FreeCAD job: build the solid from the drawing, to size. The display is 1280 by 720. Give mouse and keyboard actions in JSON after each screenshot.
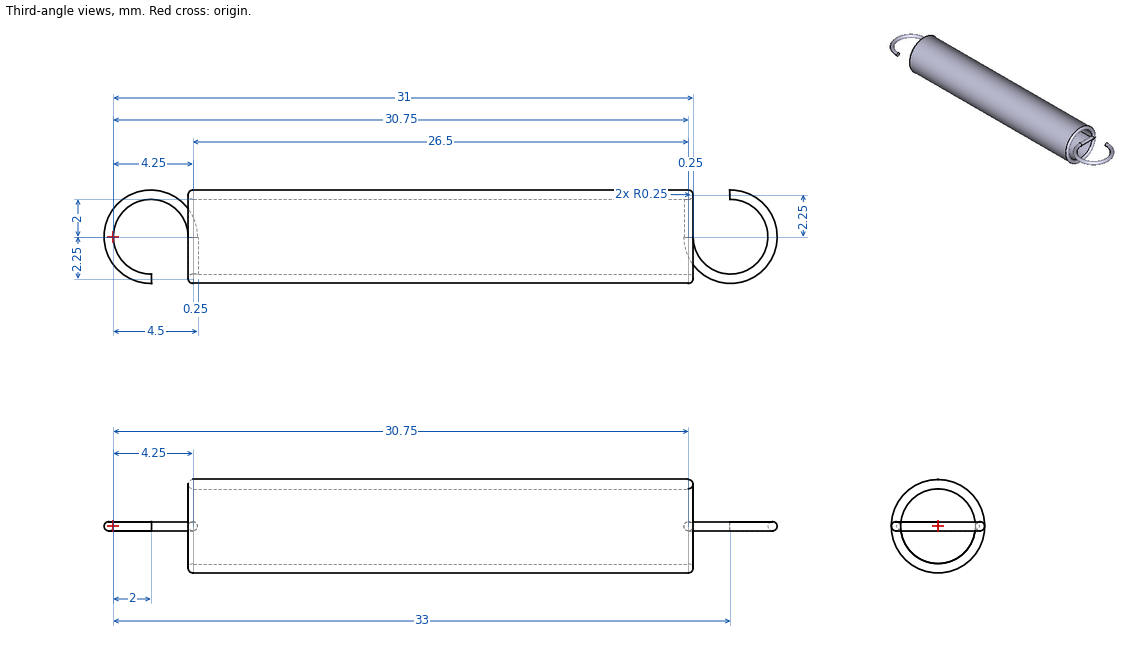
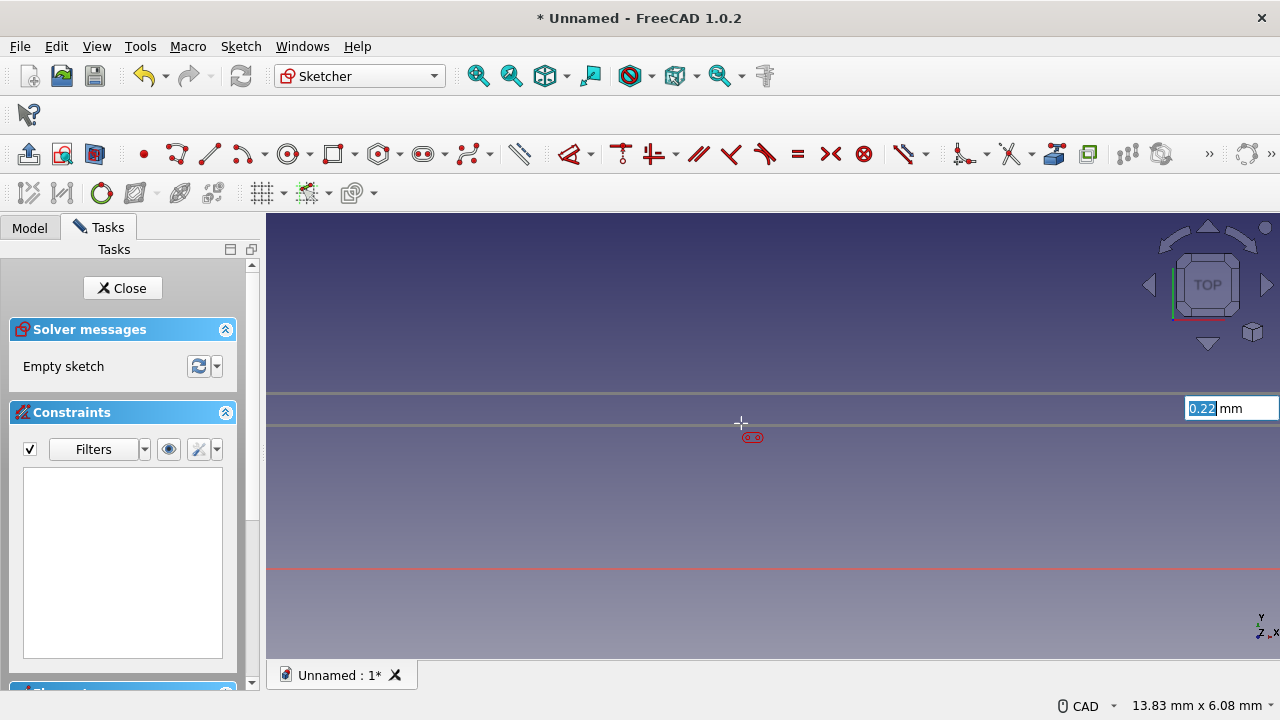
{"action": "left_click", "coordinate": [740, 422]}
{"action": "key", "text": "Escape"}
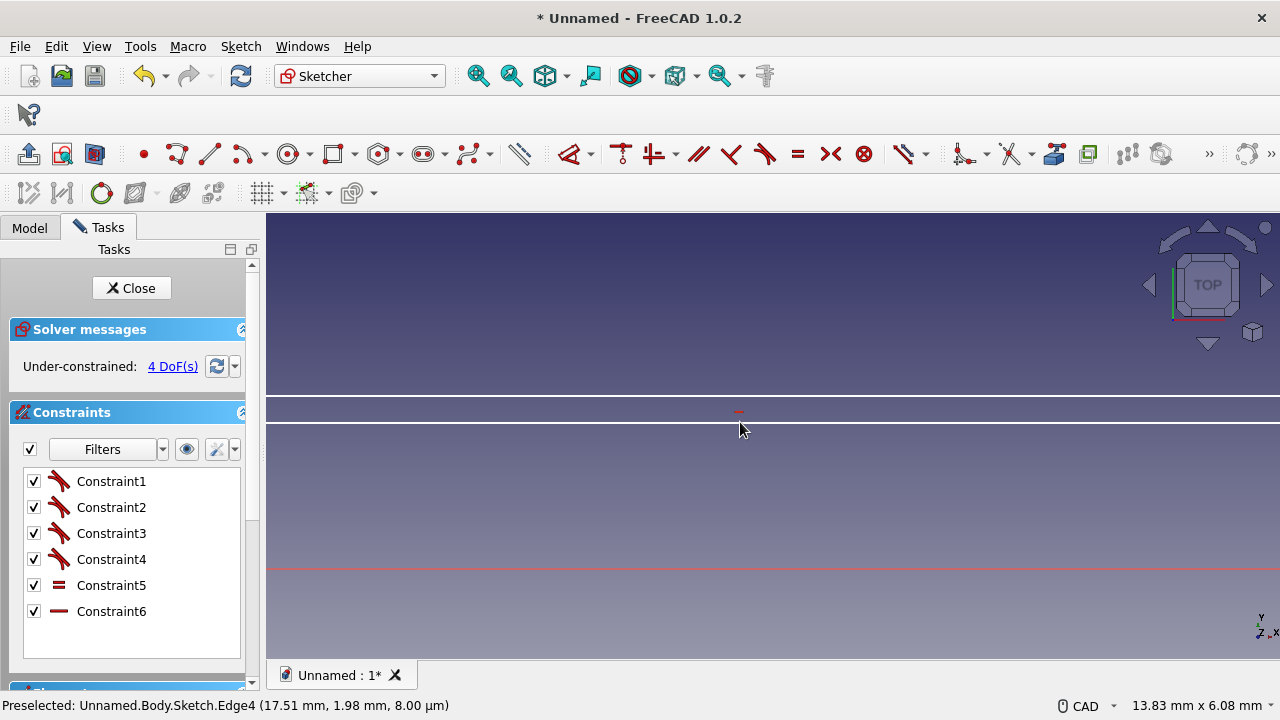
{"action": "left_click", "coordinate": [568, 154]}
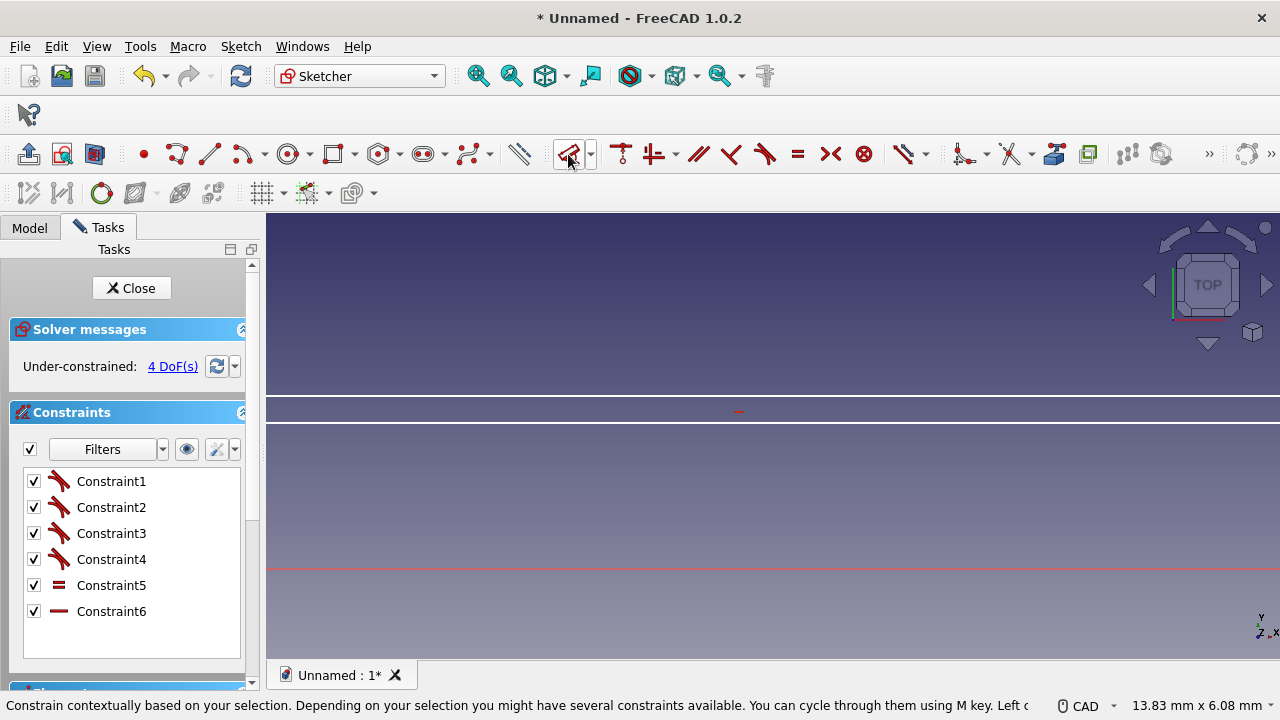
{"action": "scroll", "coordinate": [741, 423], "scroll_direction": "down", "scroll_amount": 7}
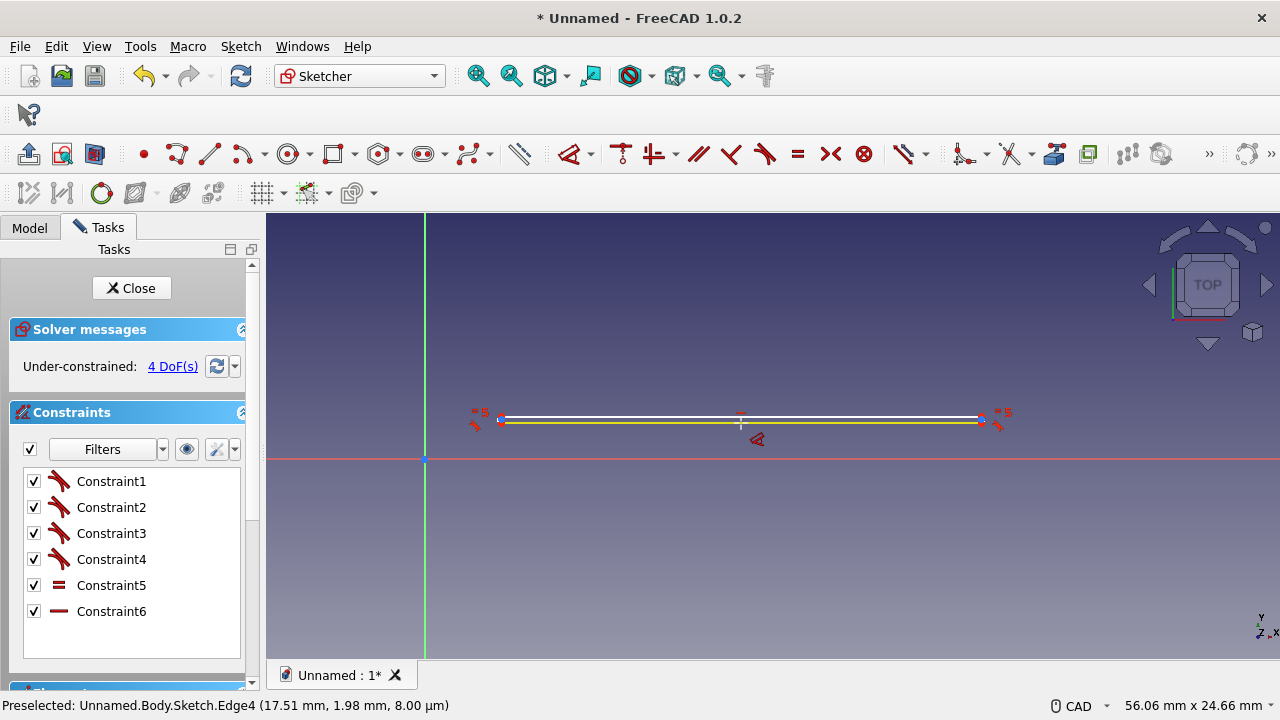
{"action": "scroll", "coordinate": [498, 418], "scroll_direction": "up", "scroll_amount": 11}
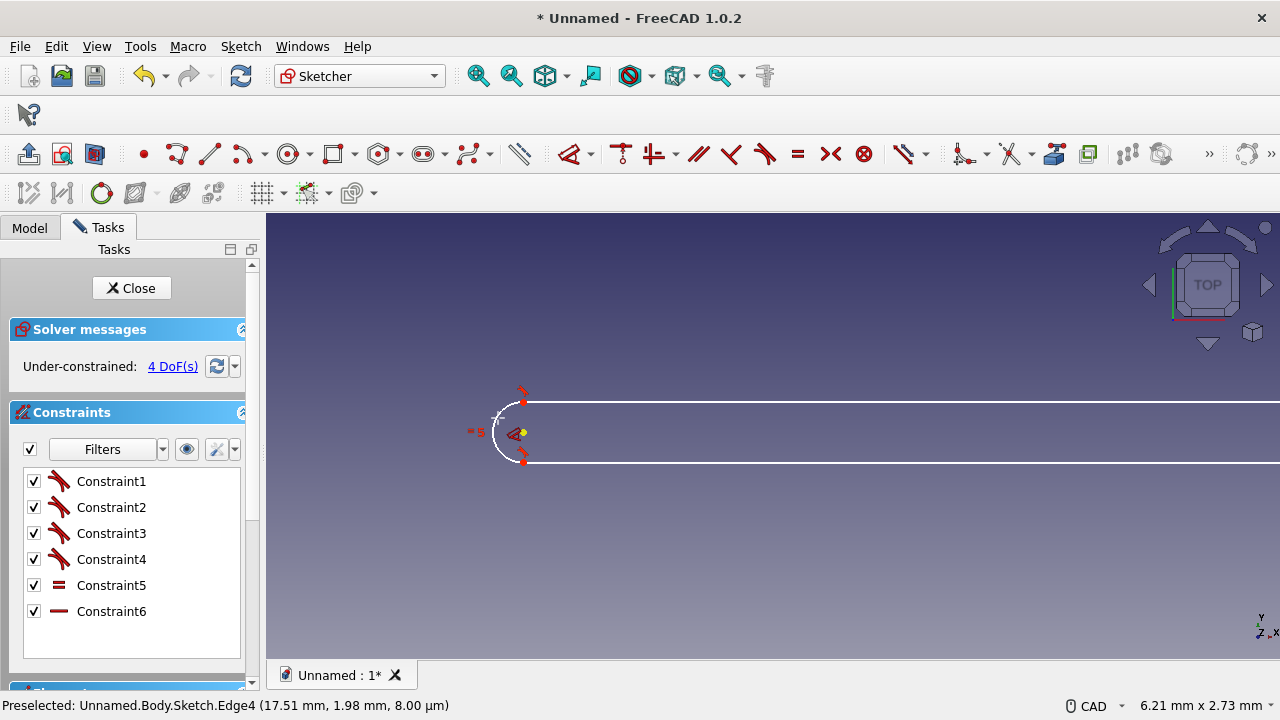
{"action": "left_click", "coordinate": [499, 415]}
{"action": "left_click", "coordinate": [473, 396]}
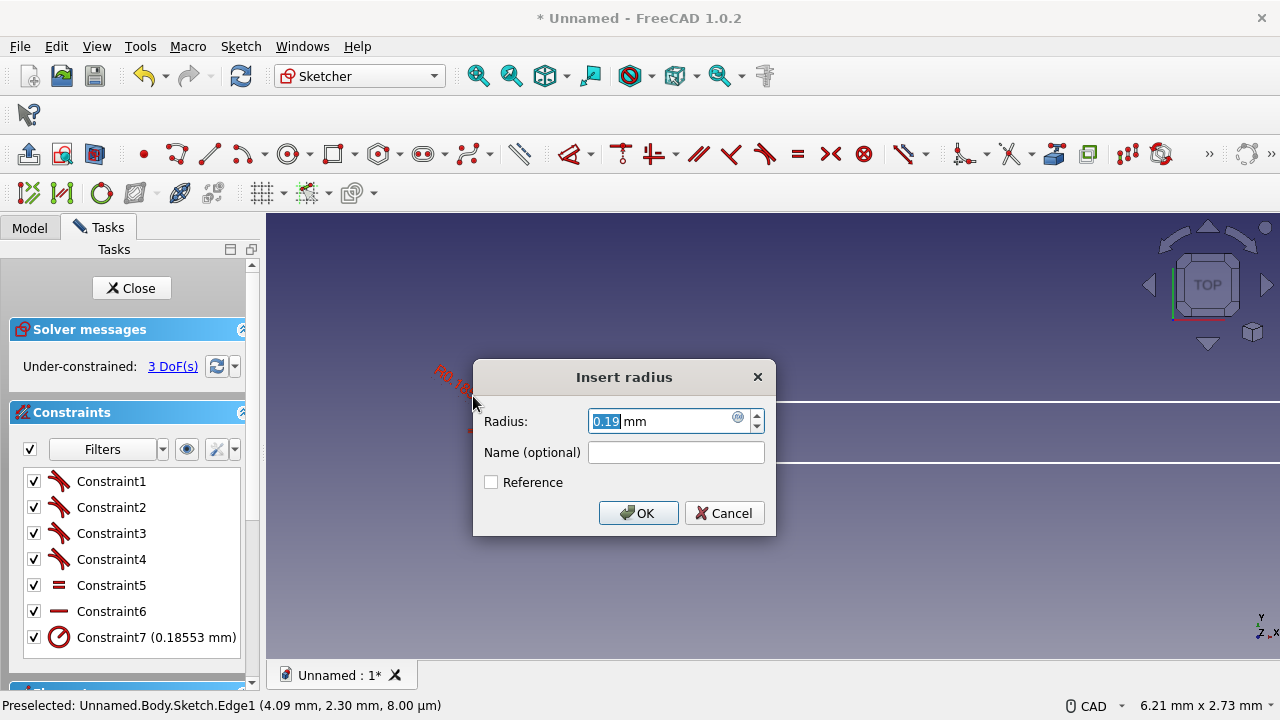
{"action": "type", "text": "0.25"}
{"action": "key", "text": "Return"}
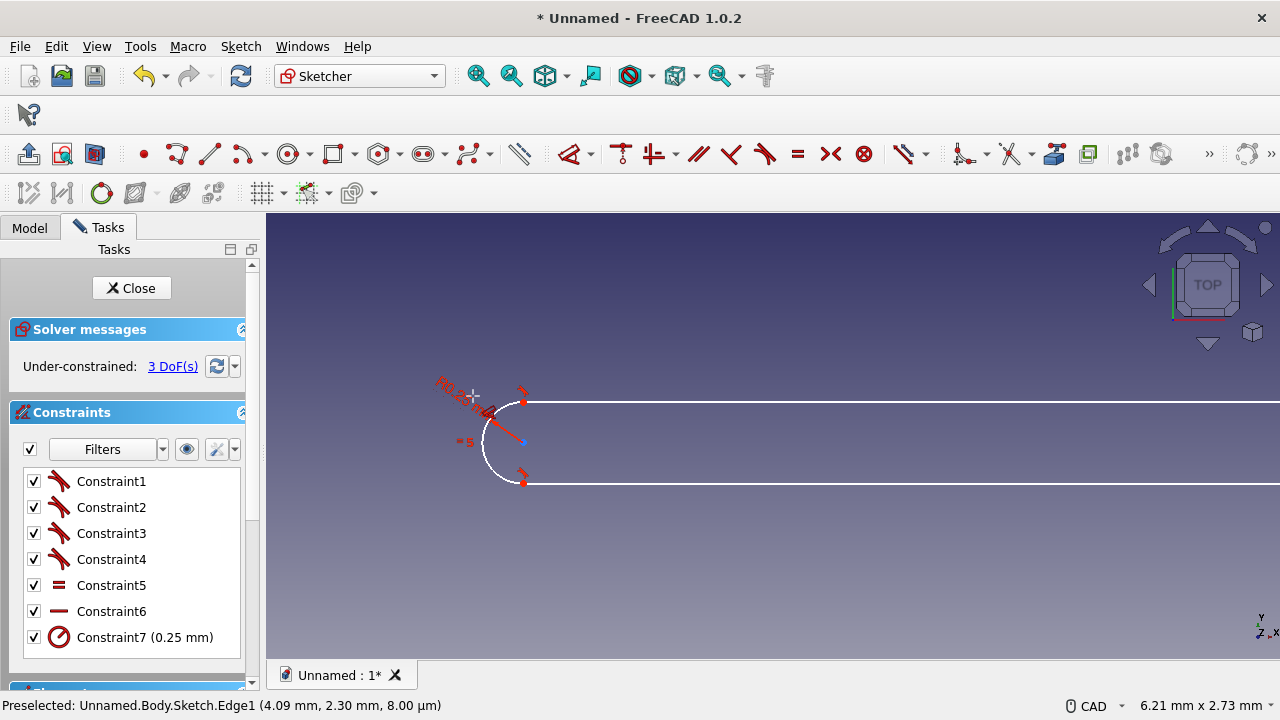
{"action": "scroll", "coordinate": [498, 418], "scroll_direction": "down", "scroll_amount": 11}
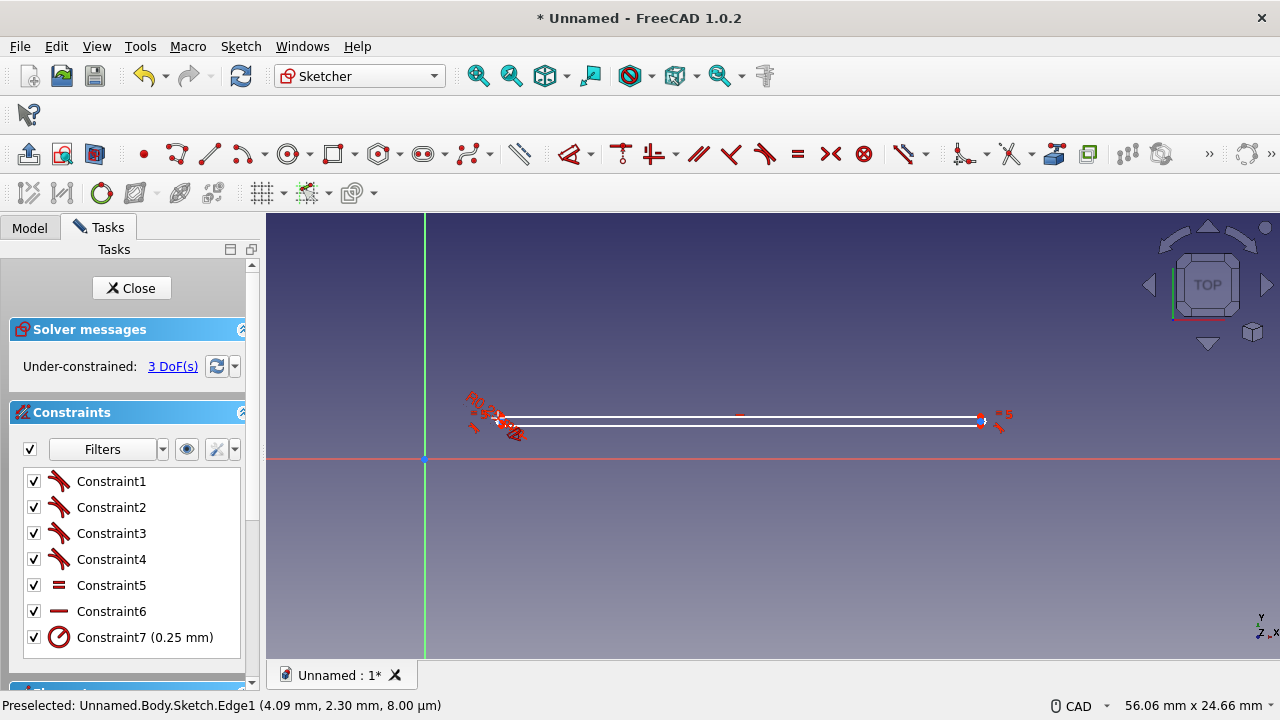
{"action": "scroll", "coordinate": [501, 426], "scroll_direction": "up", "scroll_amount": 5}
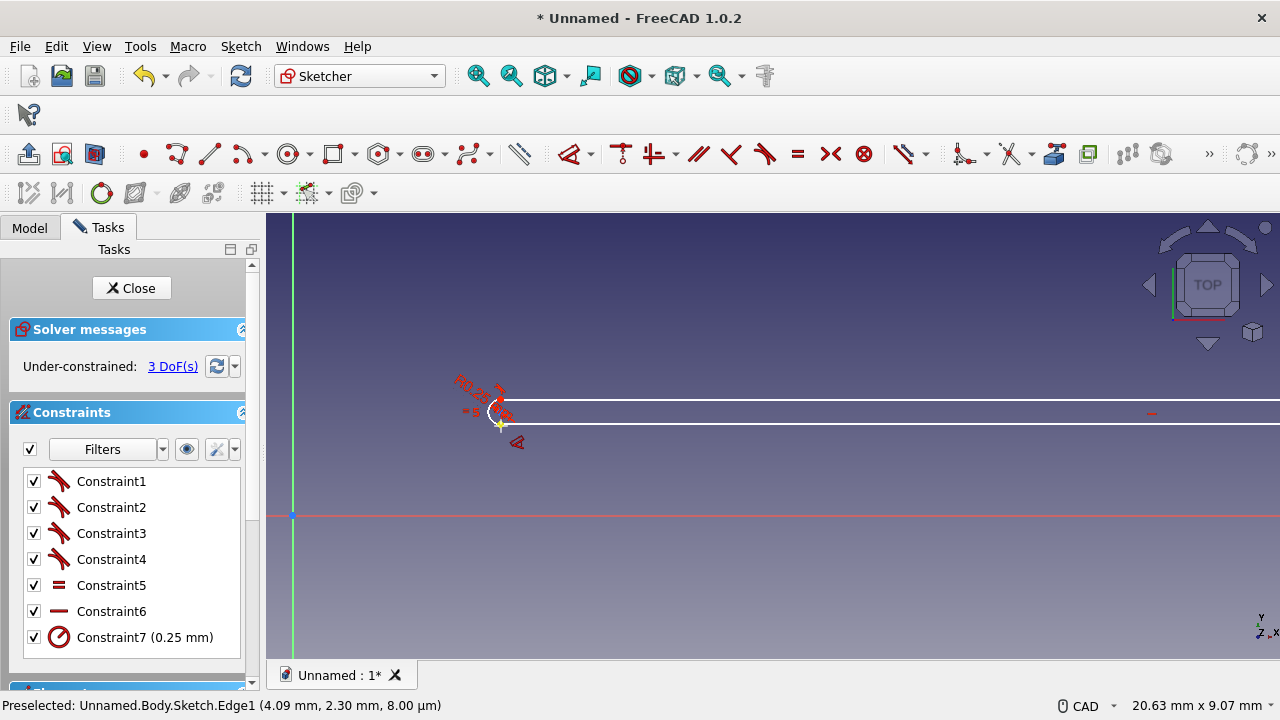
{"action": "left_click", "coordinate": [501, 424]}
{"action": "left_click", "coordinate": [535, 470]}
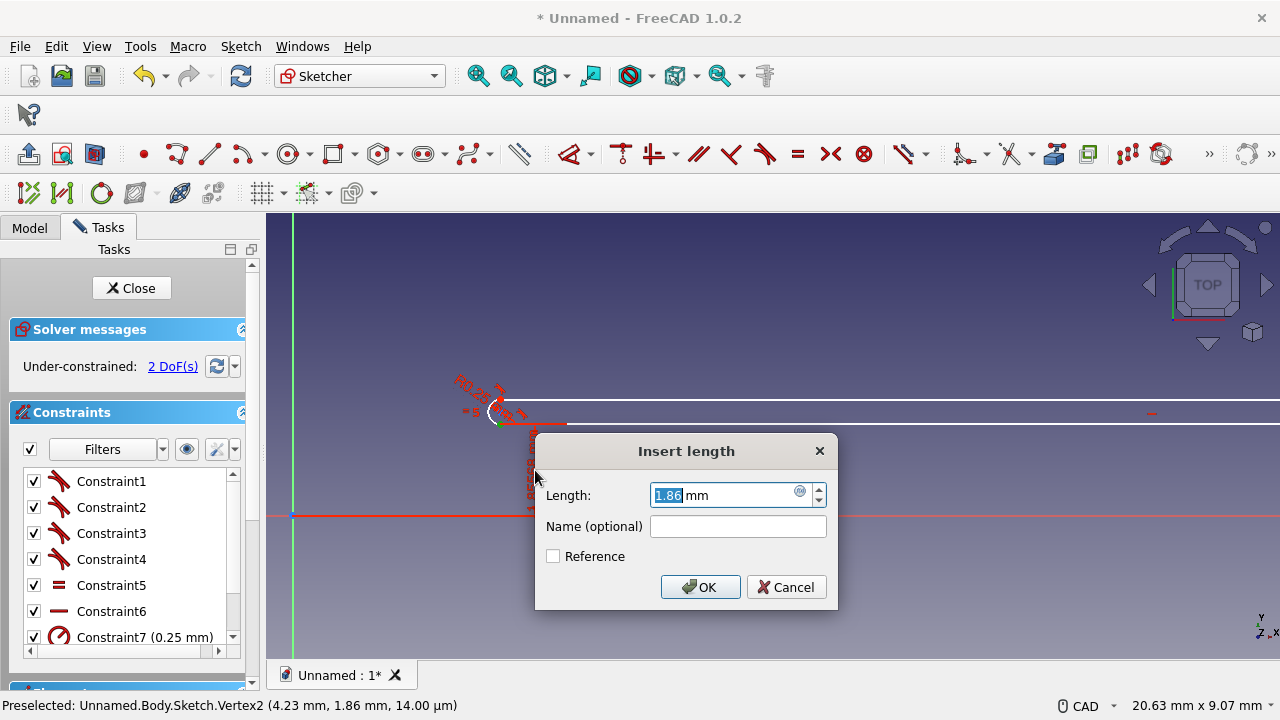
{"action": "type", "text": "2"}
{"action": "key", "text": "Return"}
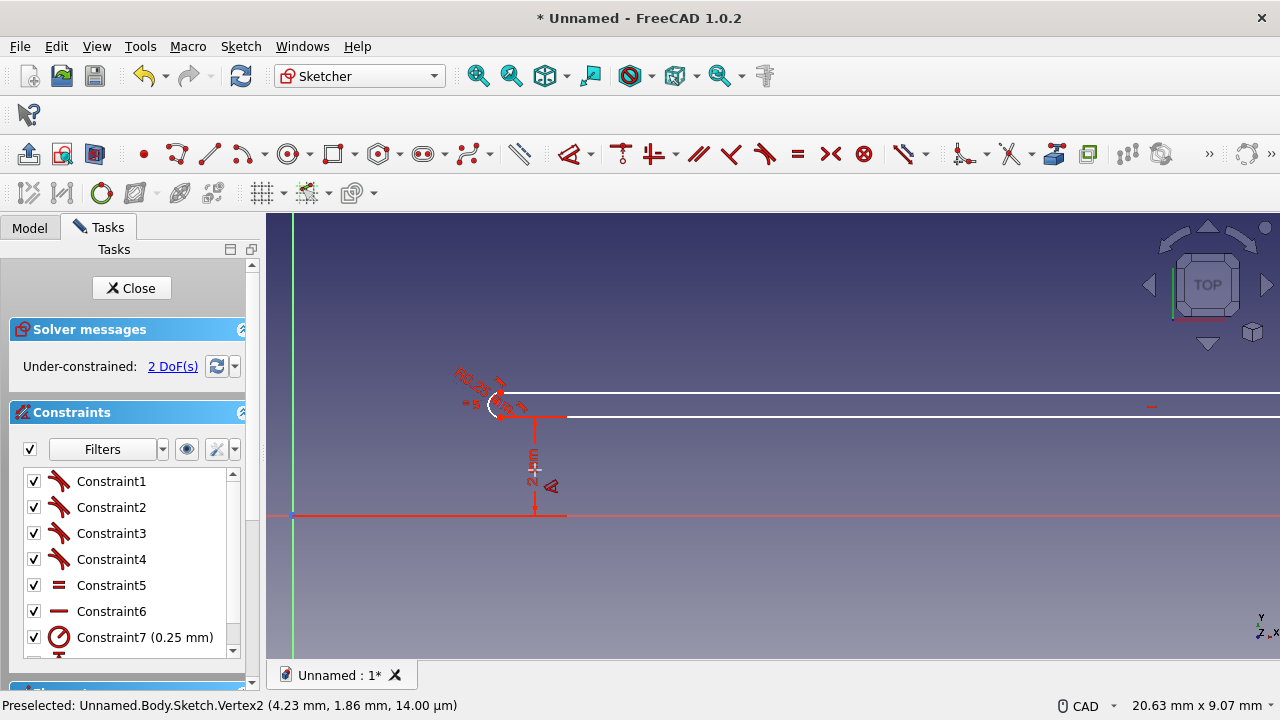
{"action": "left_click", "coordinate": [892, 393]}
{"action": "left_click", "coordinate": [808, 359]}